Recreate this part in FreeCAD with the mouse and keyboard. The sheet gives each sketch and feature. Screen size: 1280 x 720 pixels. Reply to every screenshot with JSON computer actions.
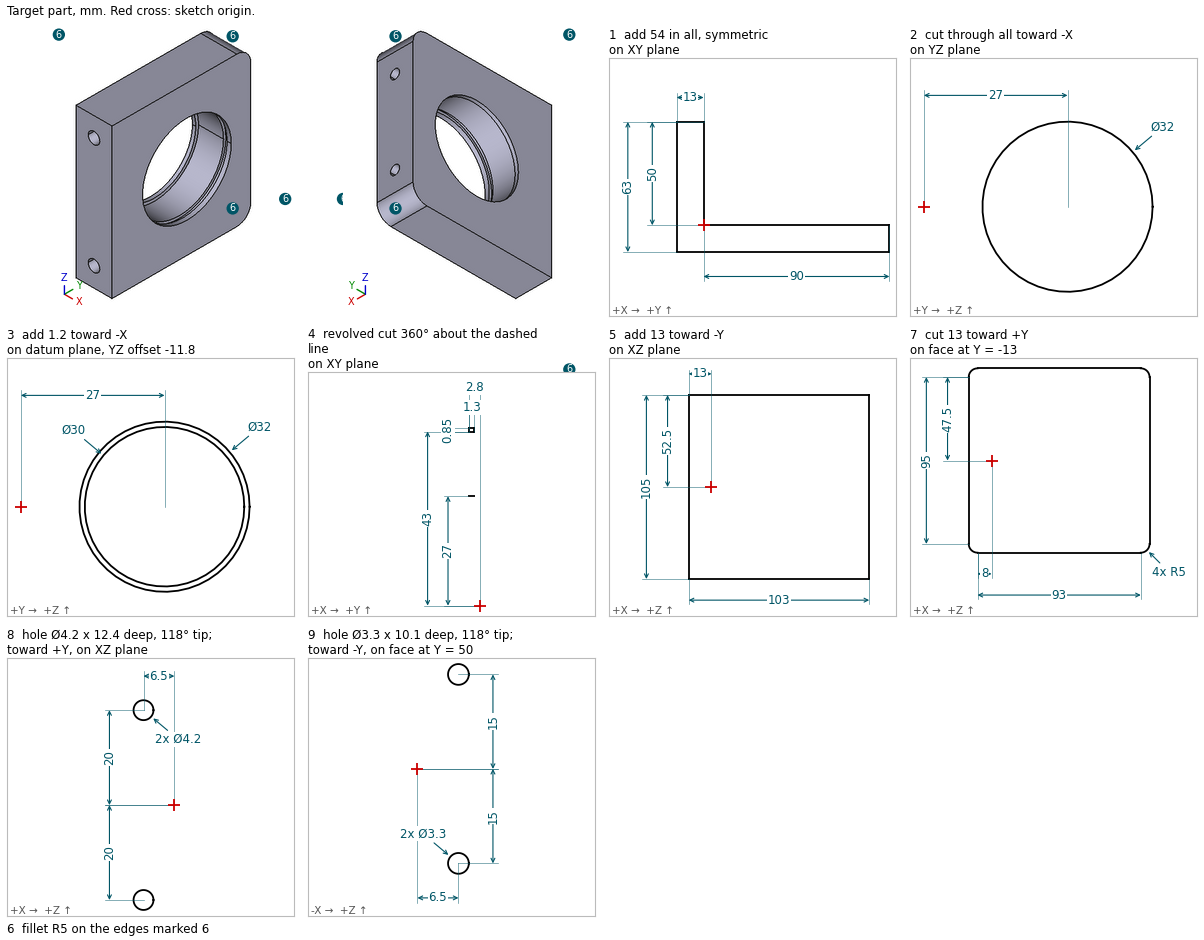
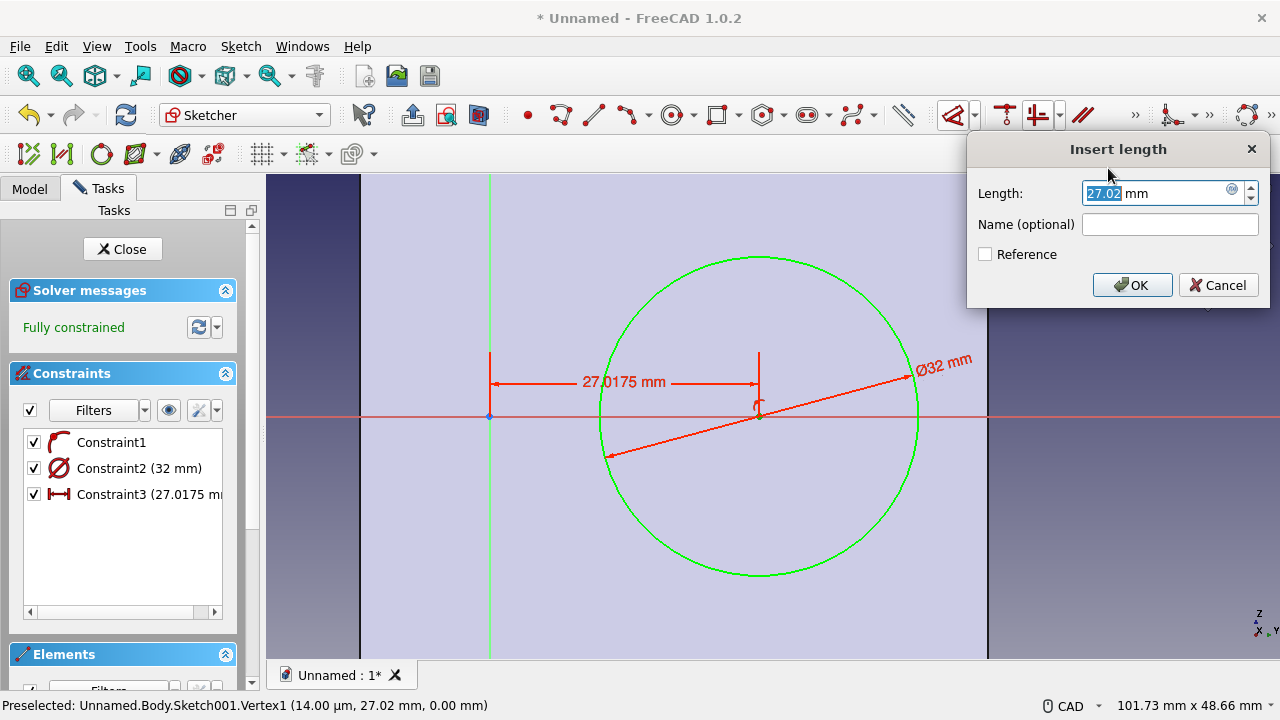
{"action": "type", "text": "27"}
{"action": "key", "text": "Return"}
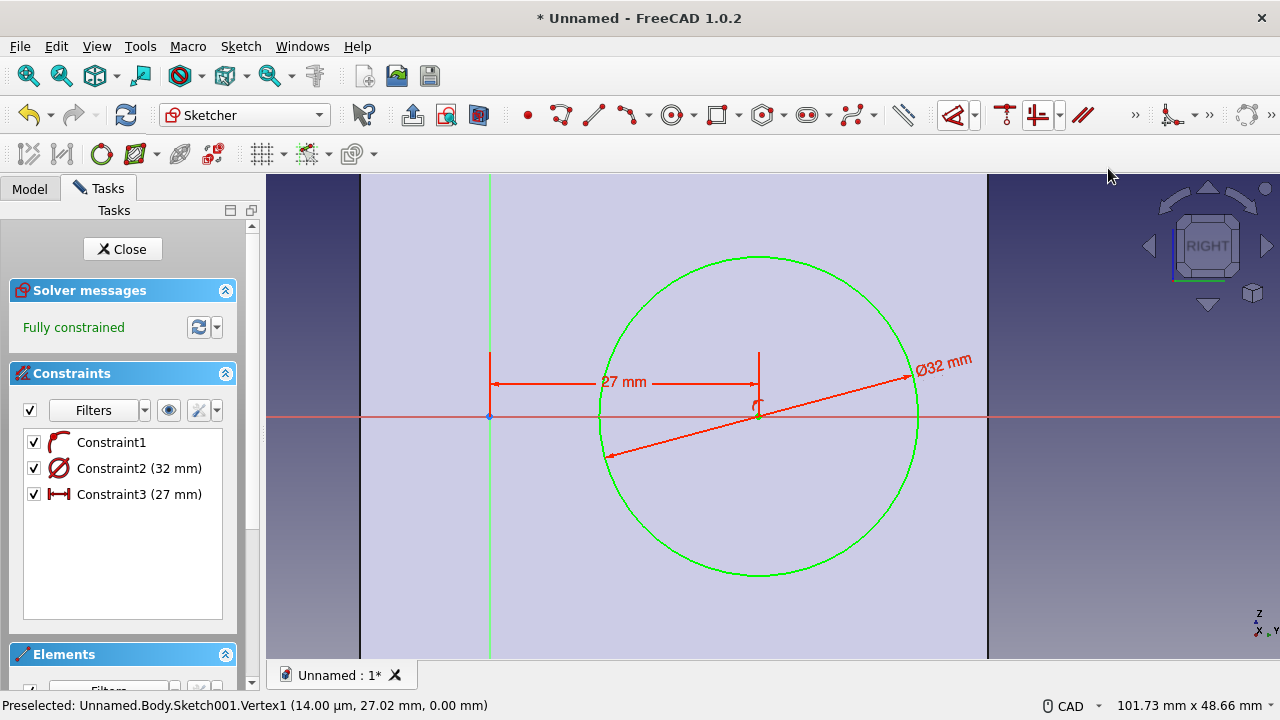
{"action": "left_click", "coordinate": [123, 249]}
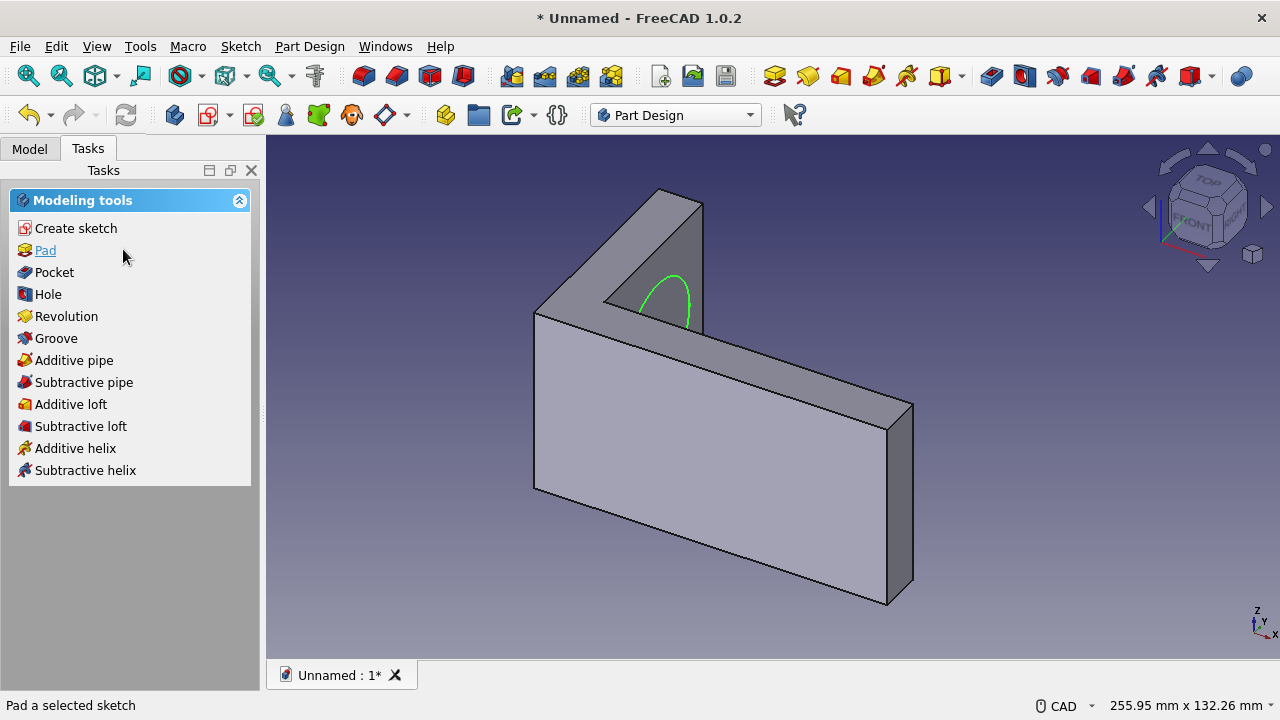
{"action": "left_click", "coordinate": [992, 76]}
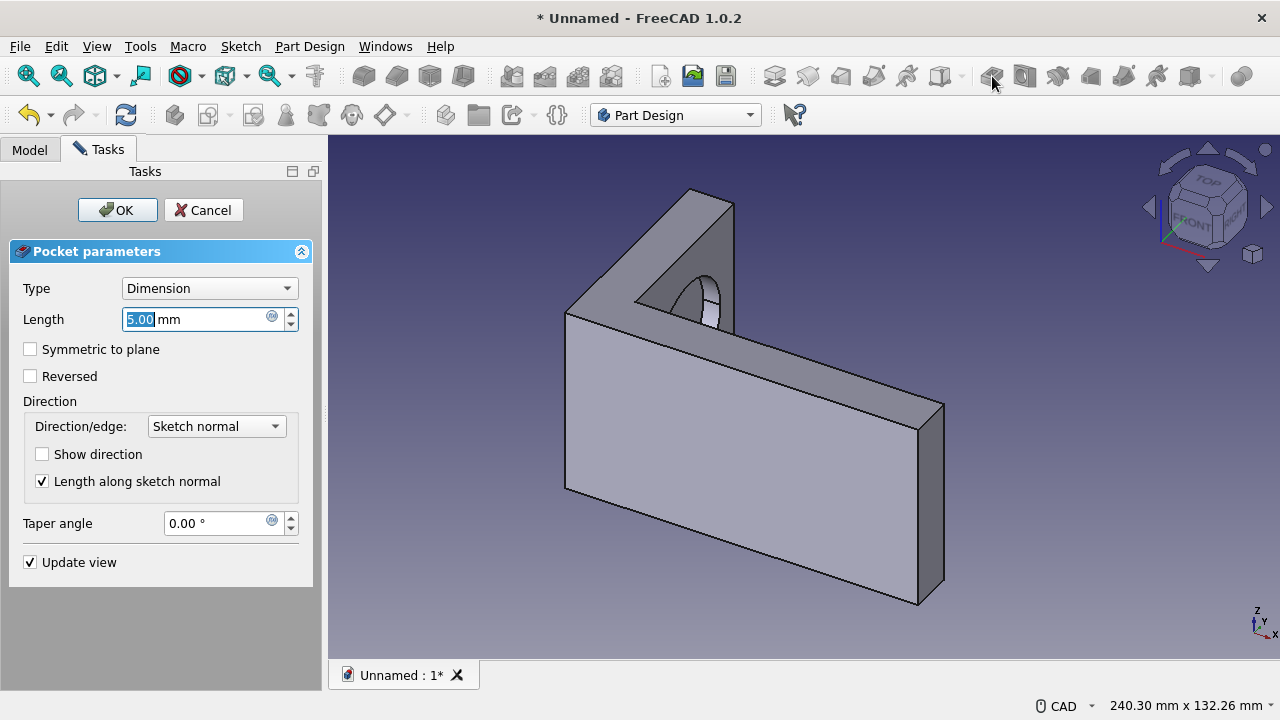
{"action": "left_click", "coordinate": [210, 288]}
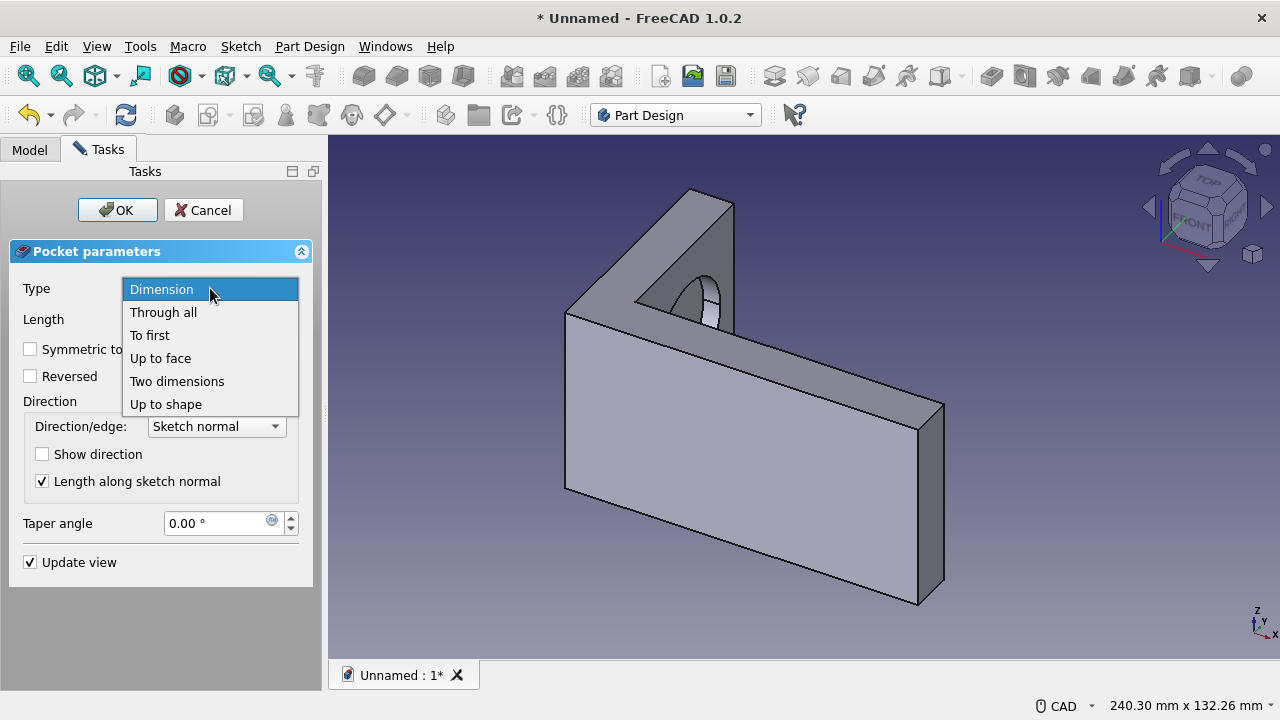
{"action": "left_click", "coordinate": [208, 312]}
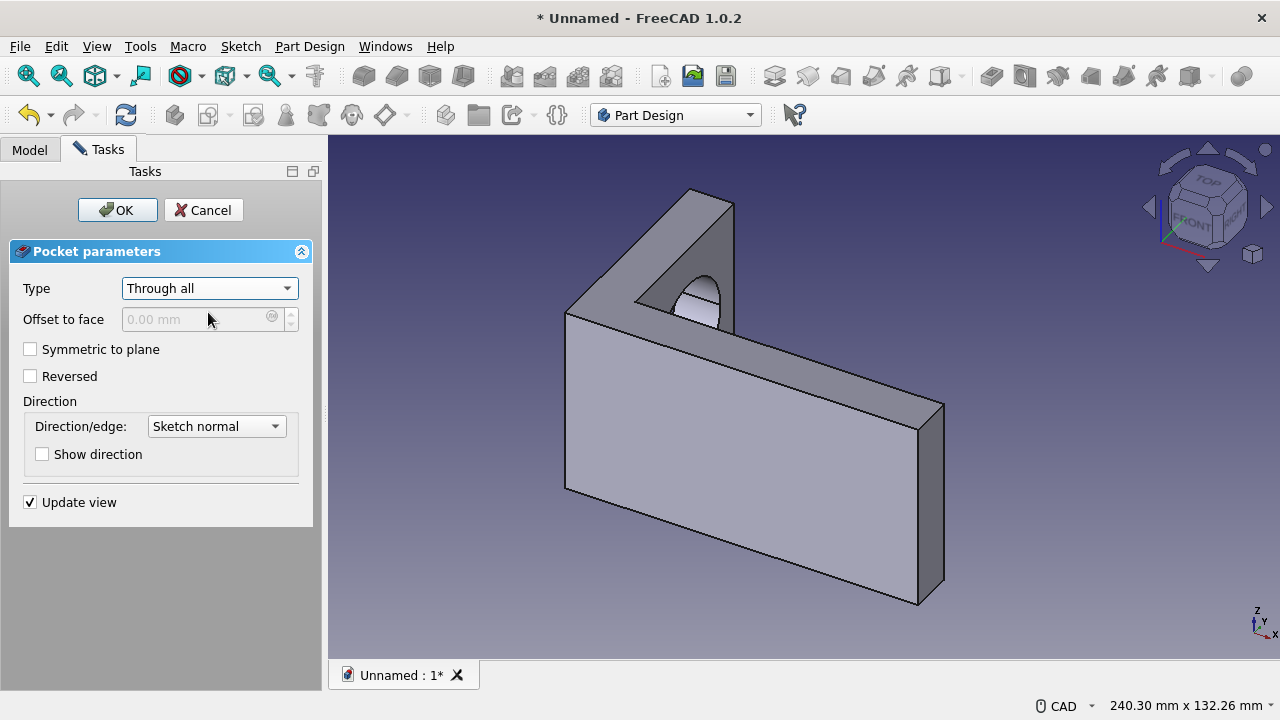
{"action": "left_click", "coordinate": [118, 210]}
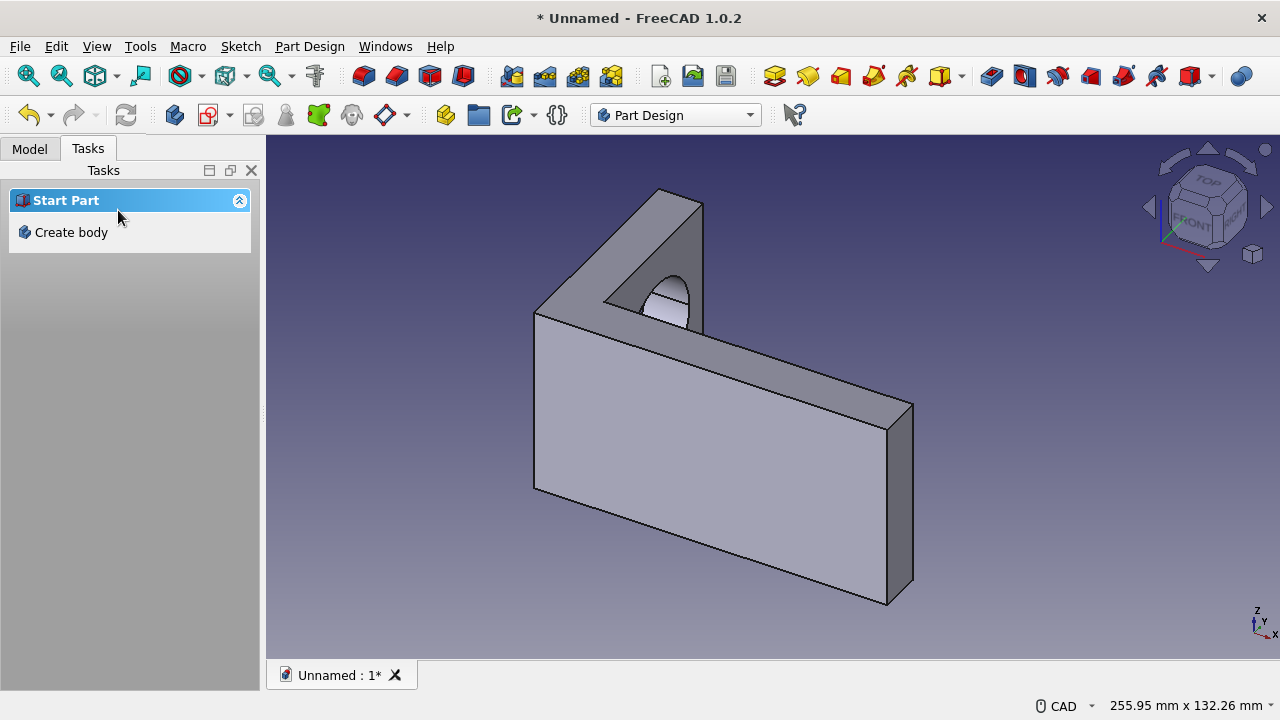
{"action": "left_click", "coordinate": [30, 148]}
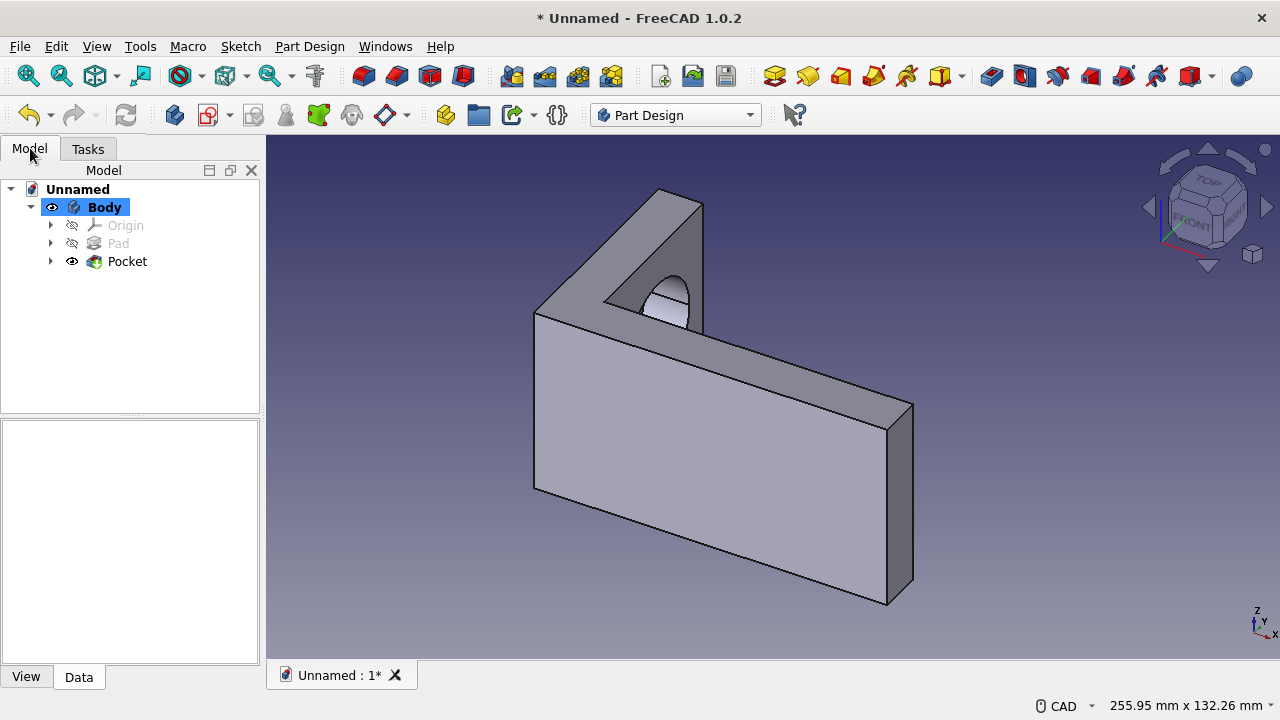
{"action": "left_click", "coordinate": [51, 225]}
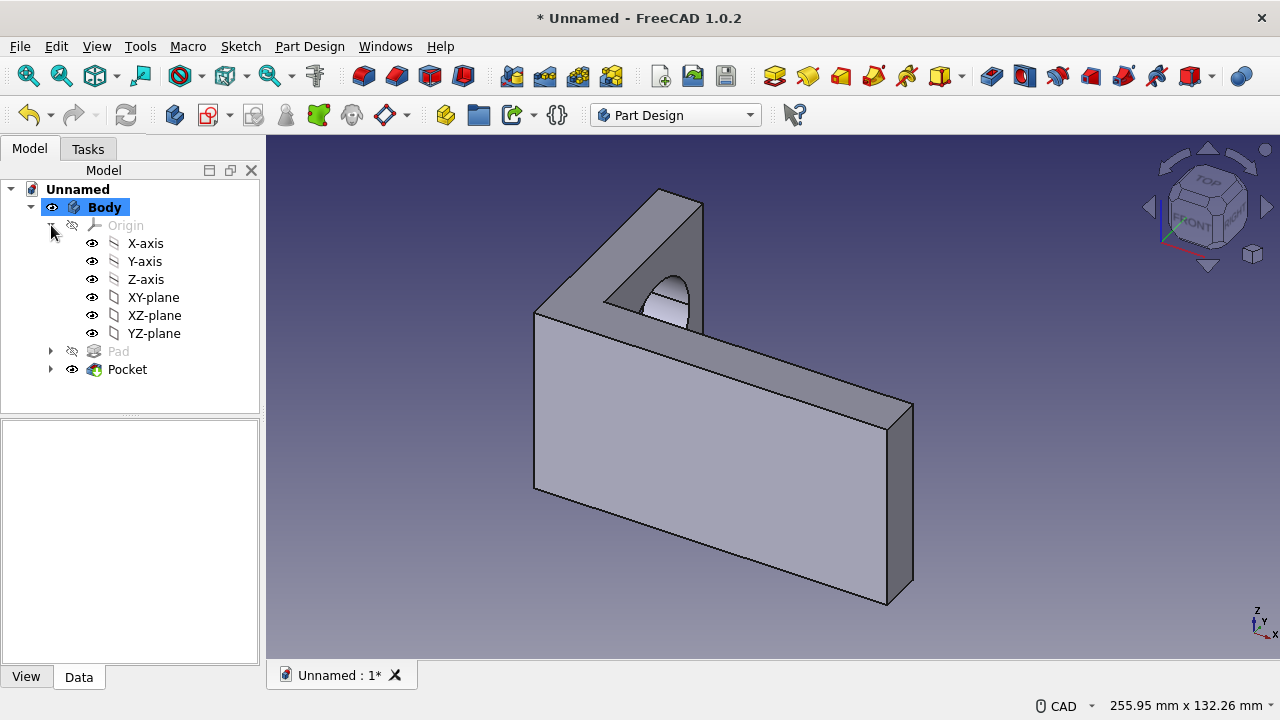
{"action": "left_click", "coordinate": [137, 333]}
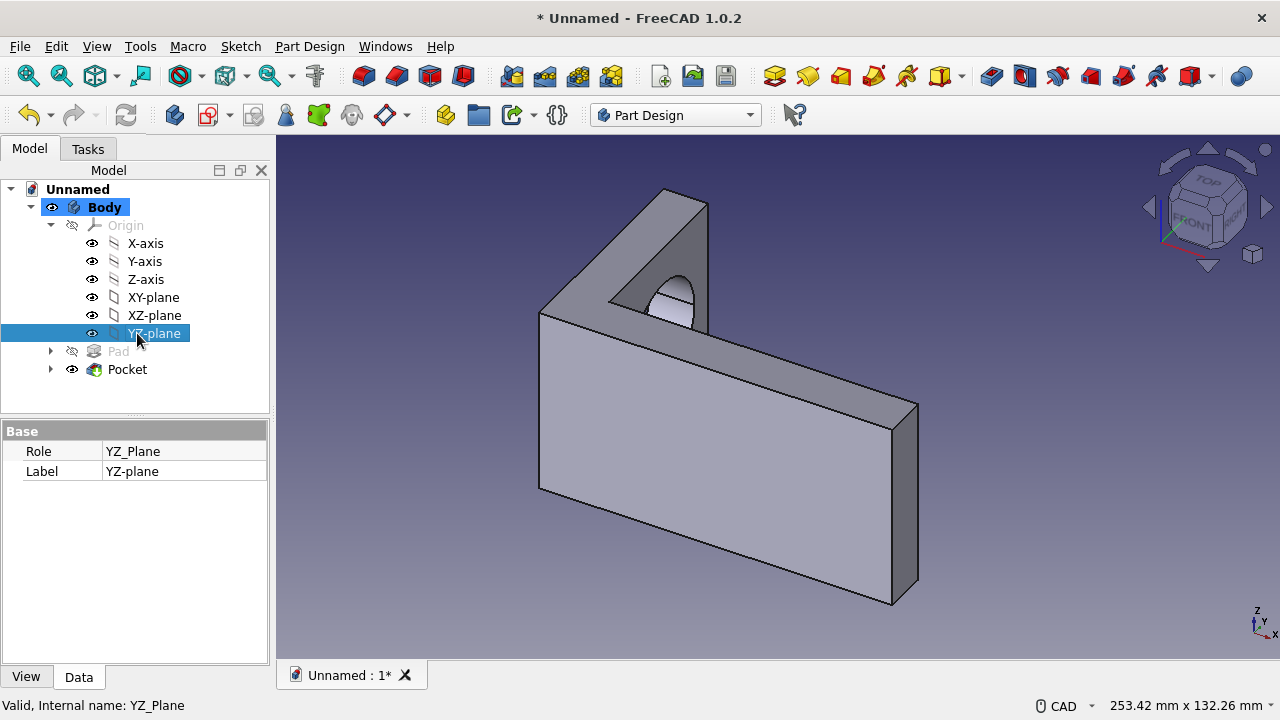
{"action": "left_click", "coordinate": [384, 116]}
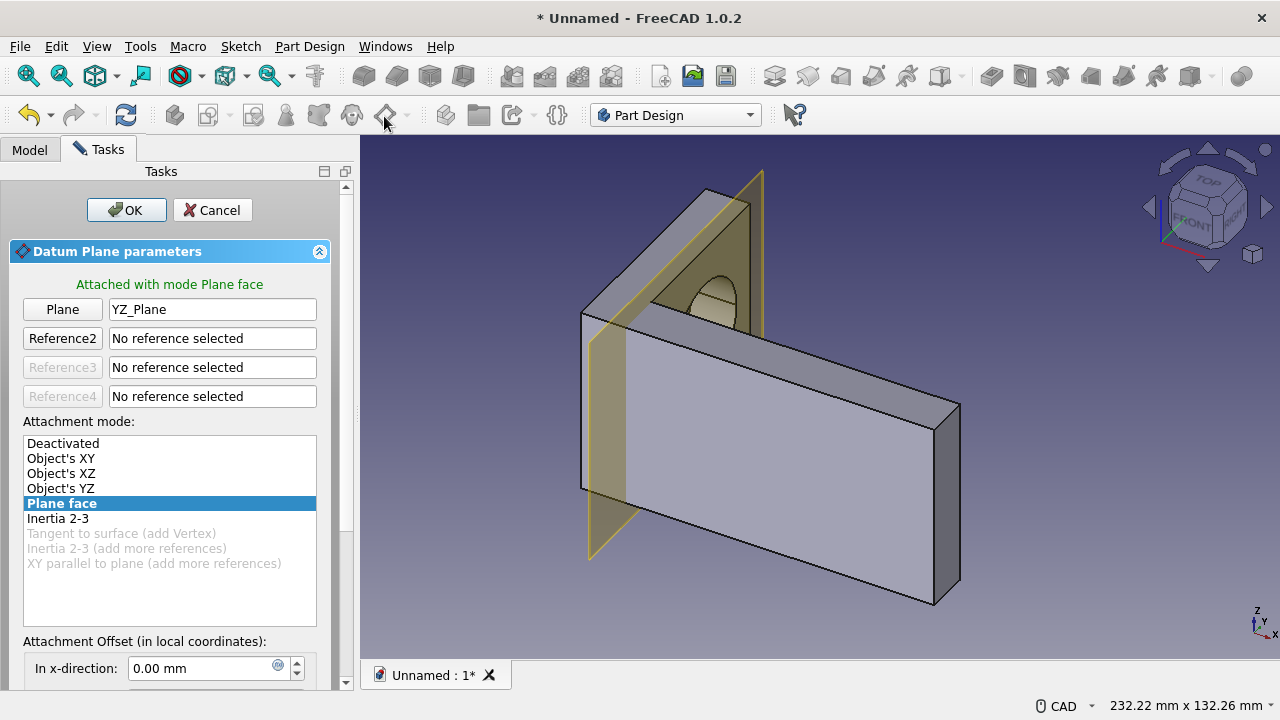
{"action": "scroll", "coordinate": [346, 436], "scroll_direction": "down", "scroll_amount": 2}